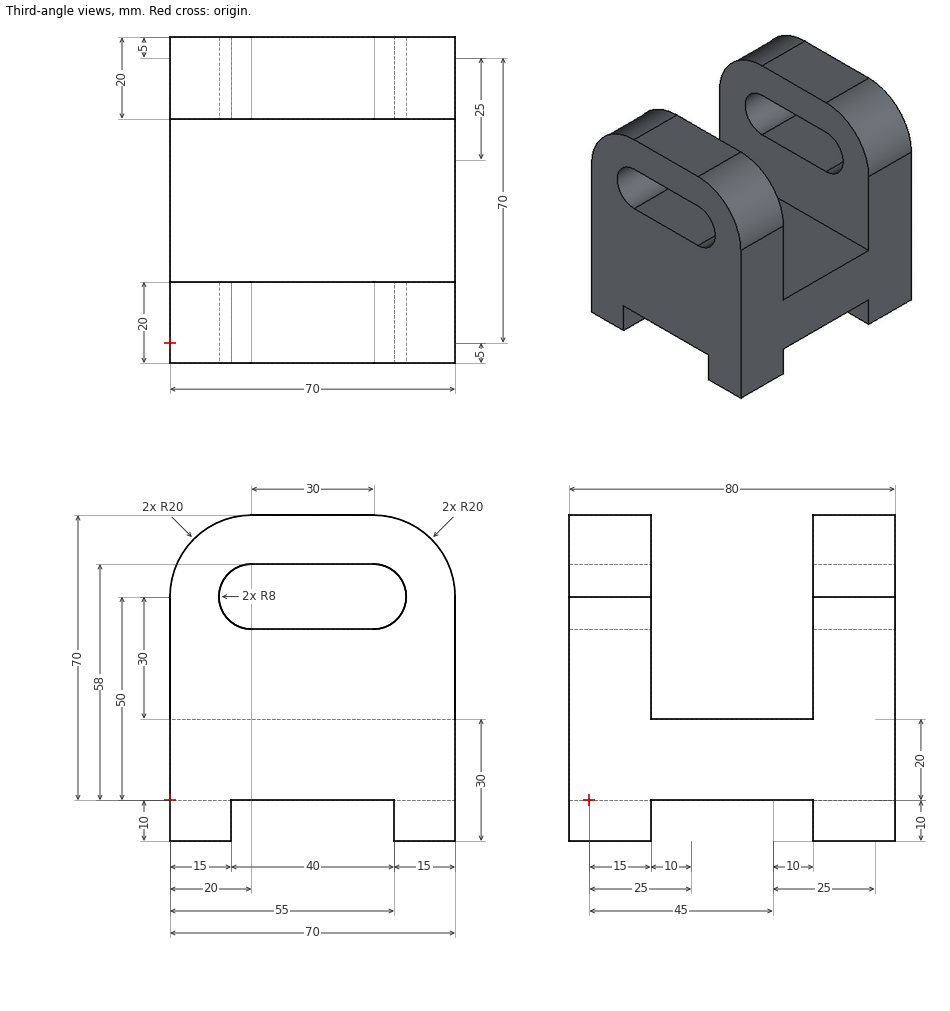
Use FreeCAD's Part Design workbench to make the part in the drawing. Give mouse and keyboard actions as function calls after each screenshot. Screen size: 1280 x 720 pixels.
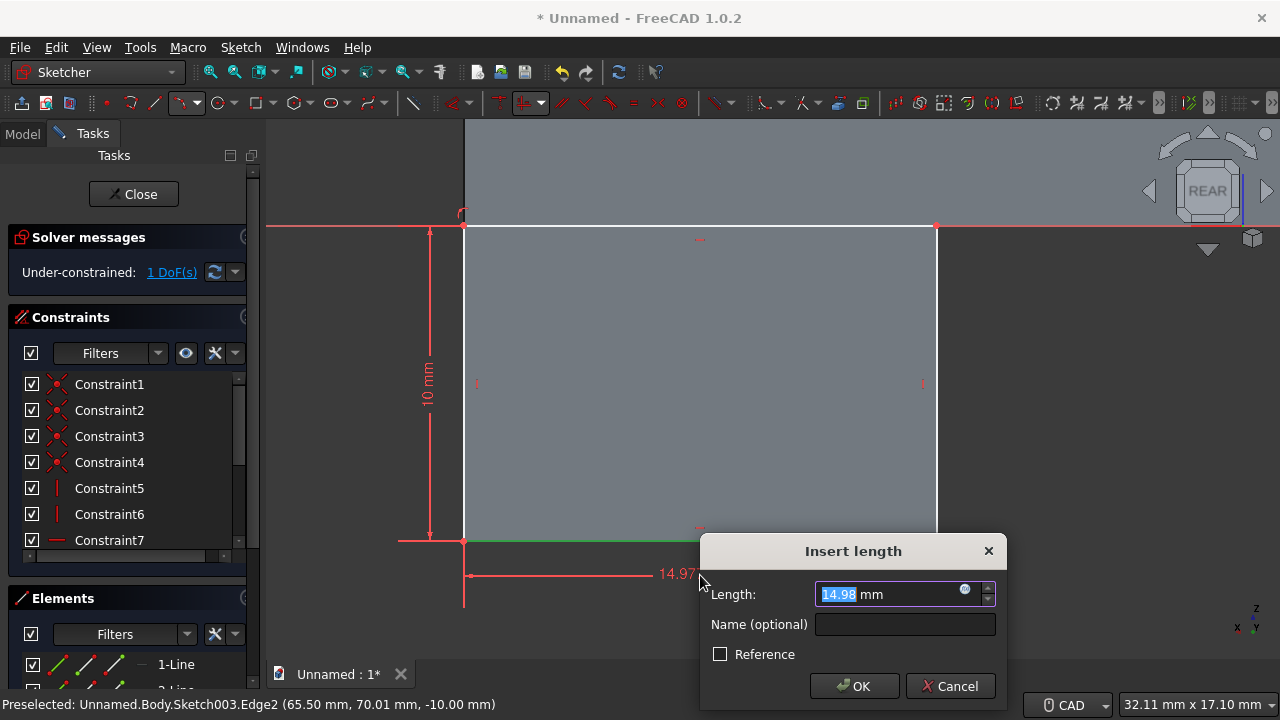
text(15)
key(Return)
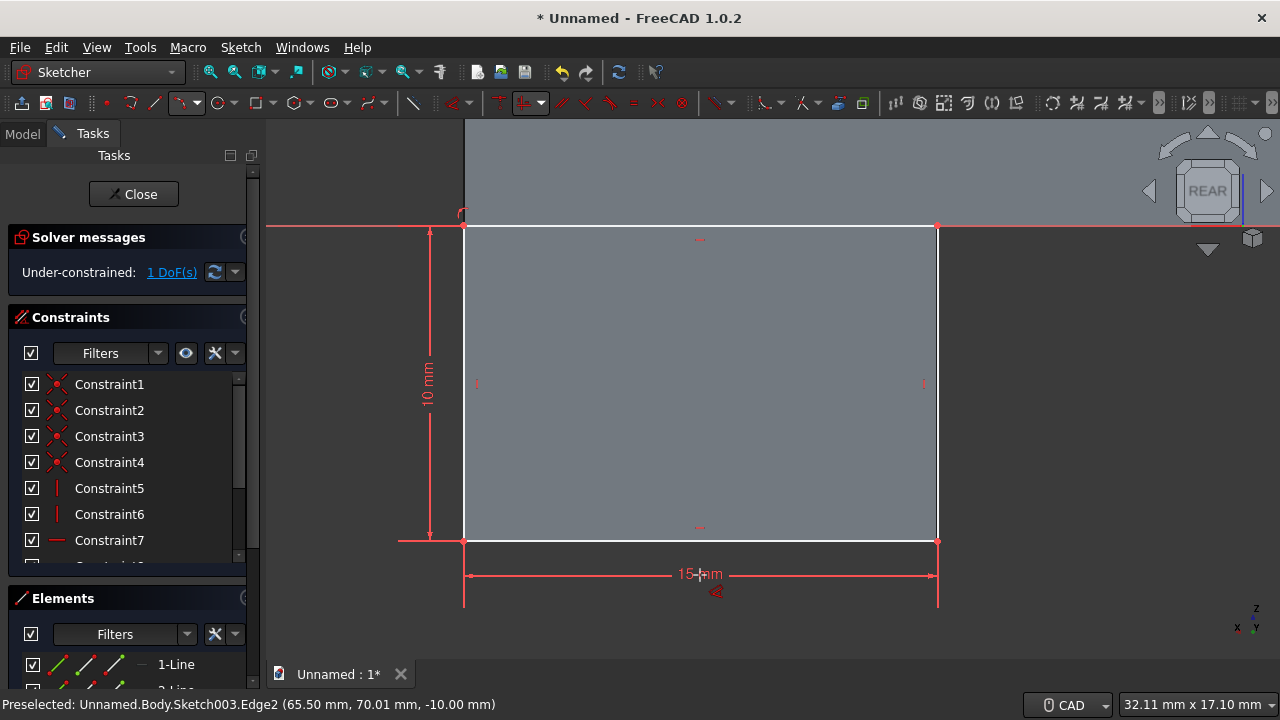
click(464, 226)
click(789, 192)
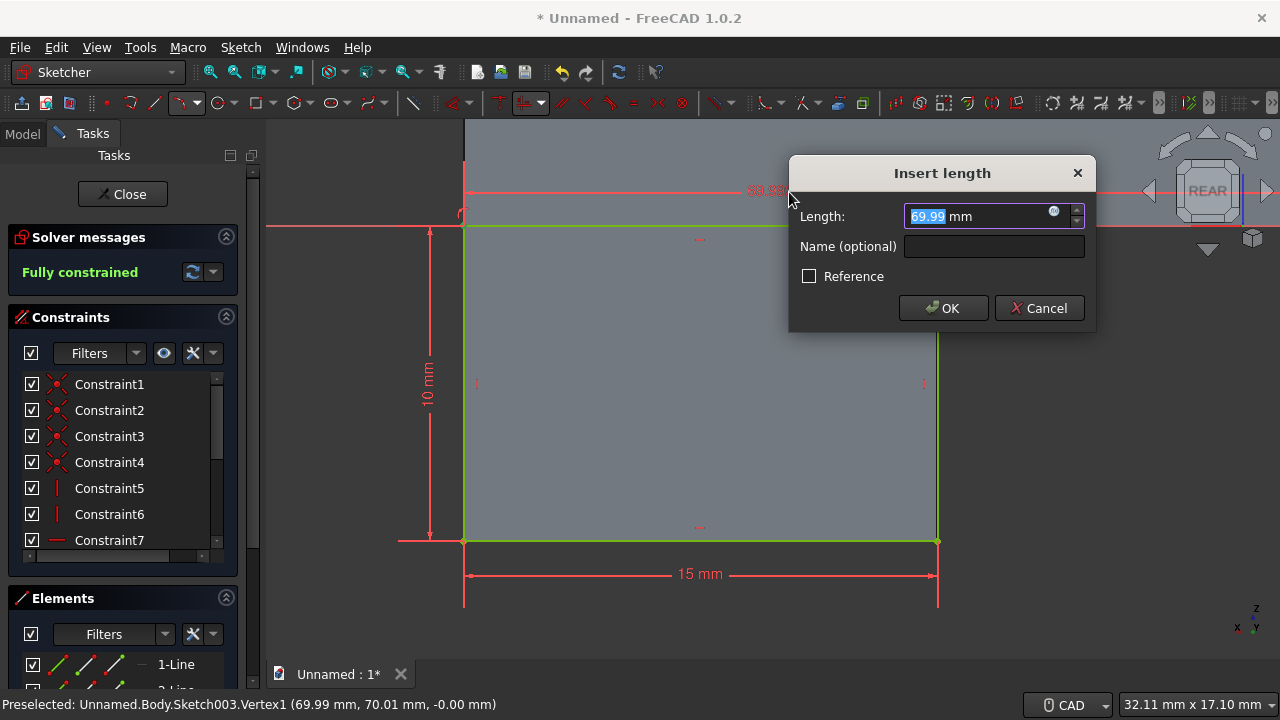
text(70)
key(Return)
key(Escape)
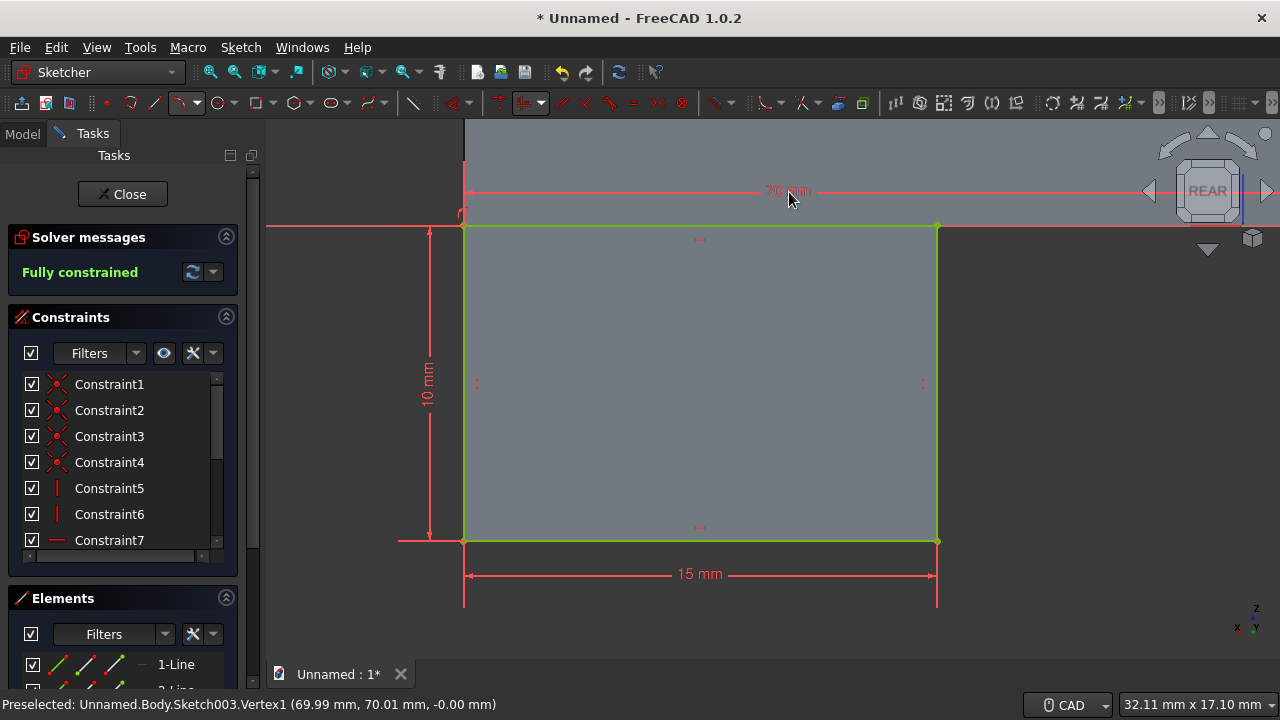
click(123, 194)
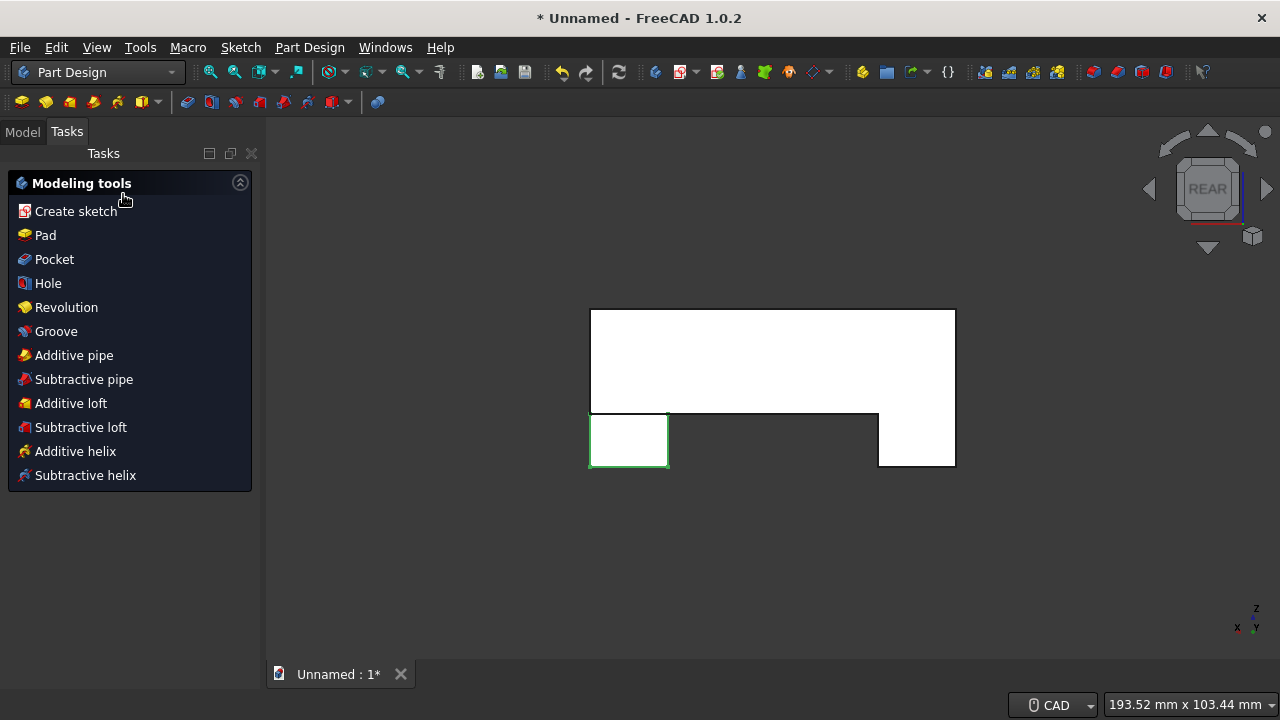
click(22, 102)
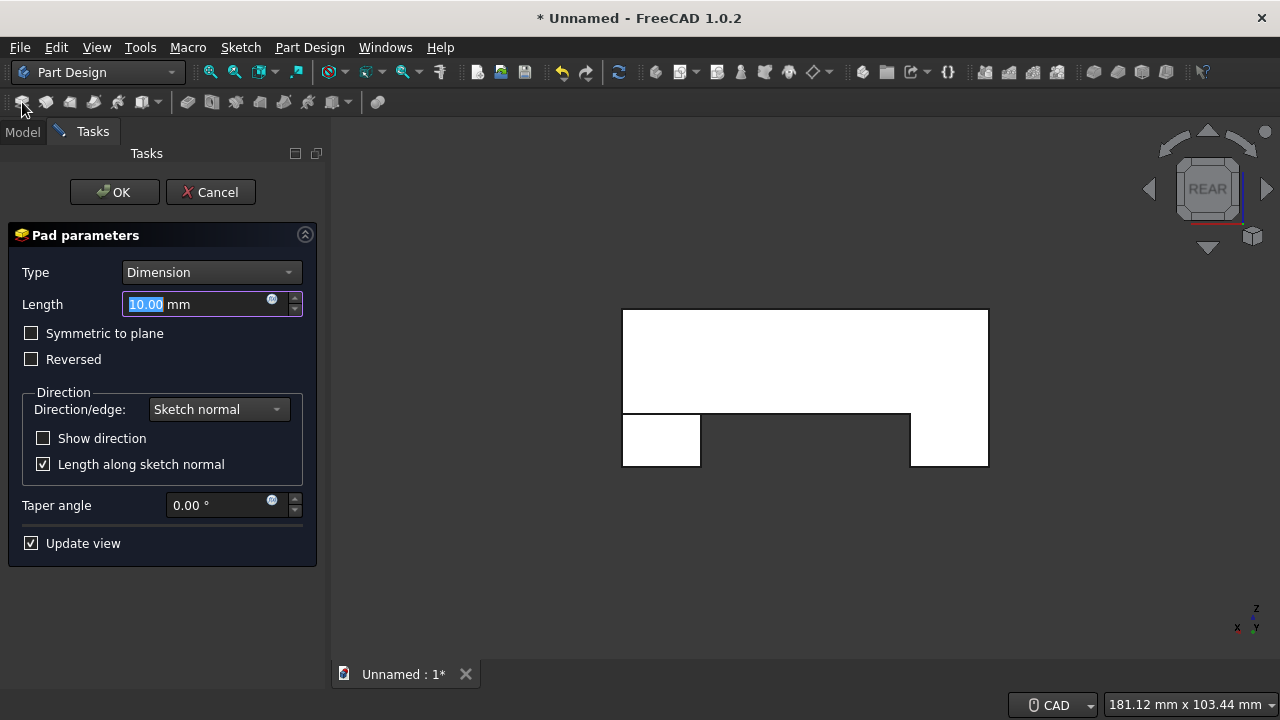
text(25)
key(Tab)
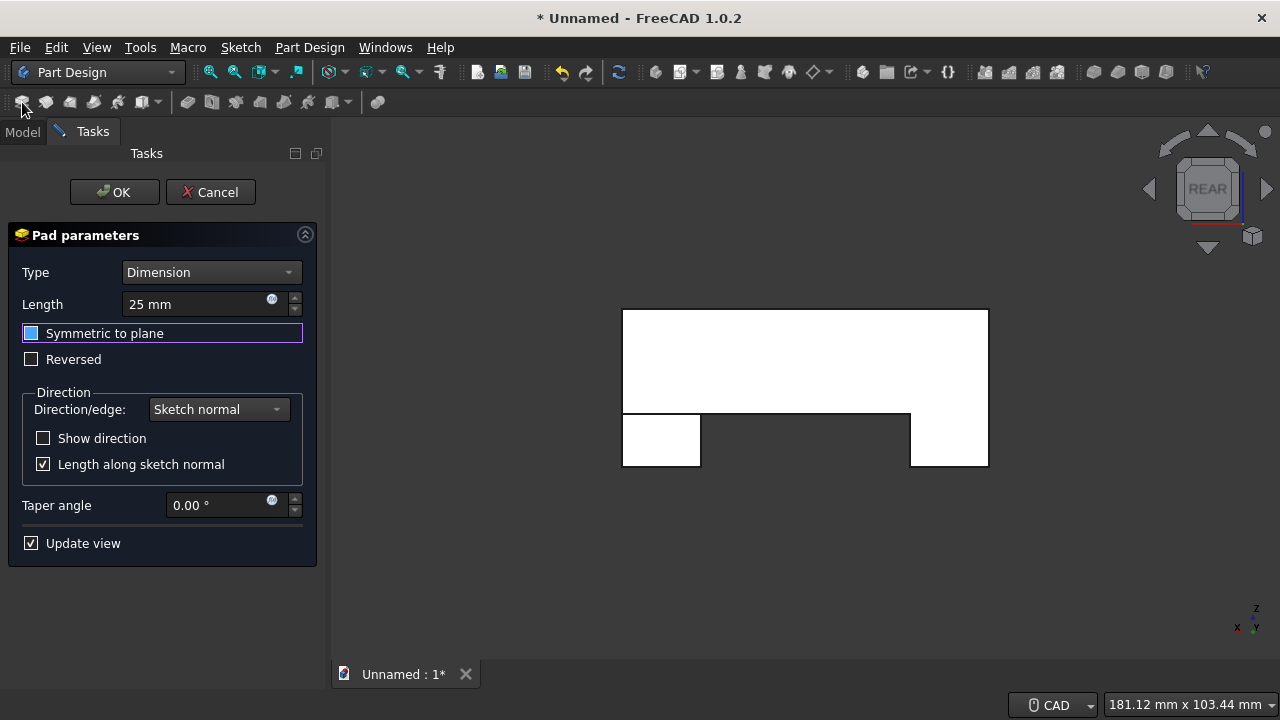
click(30, 359)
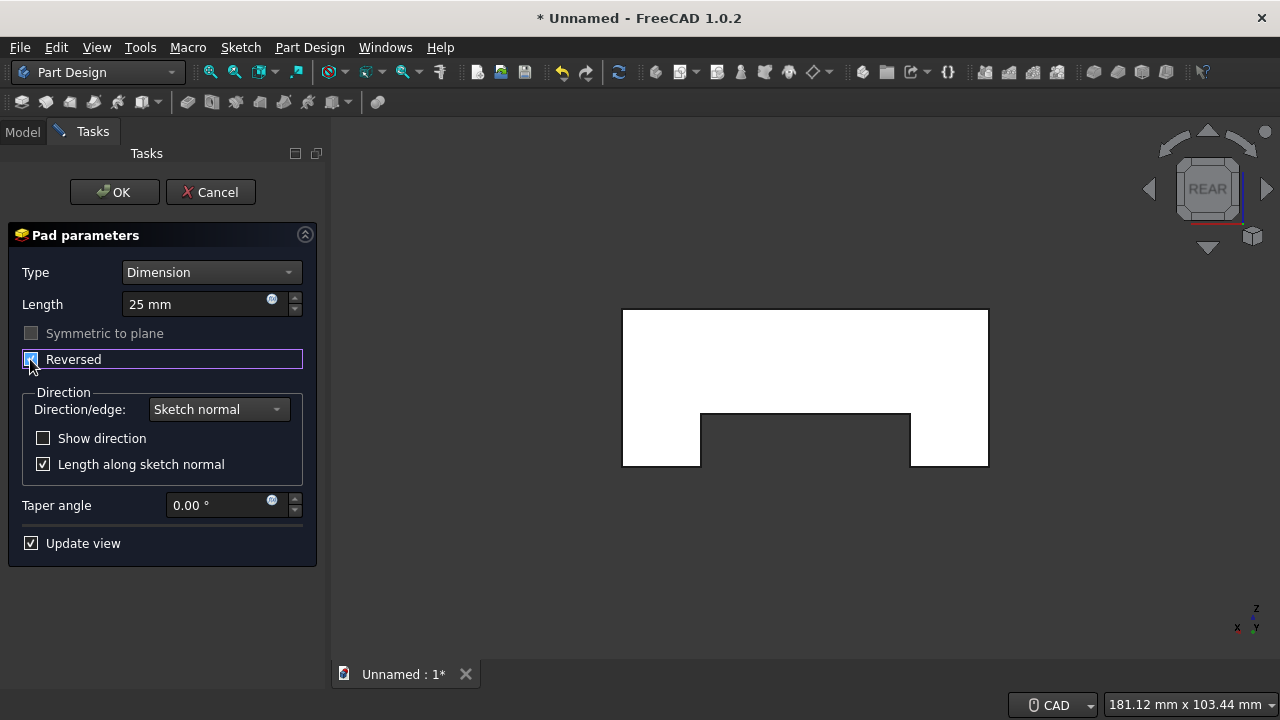
click(115, 192)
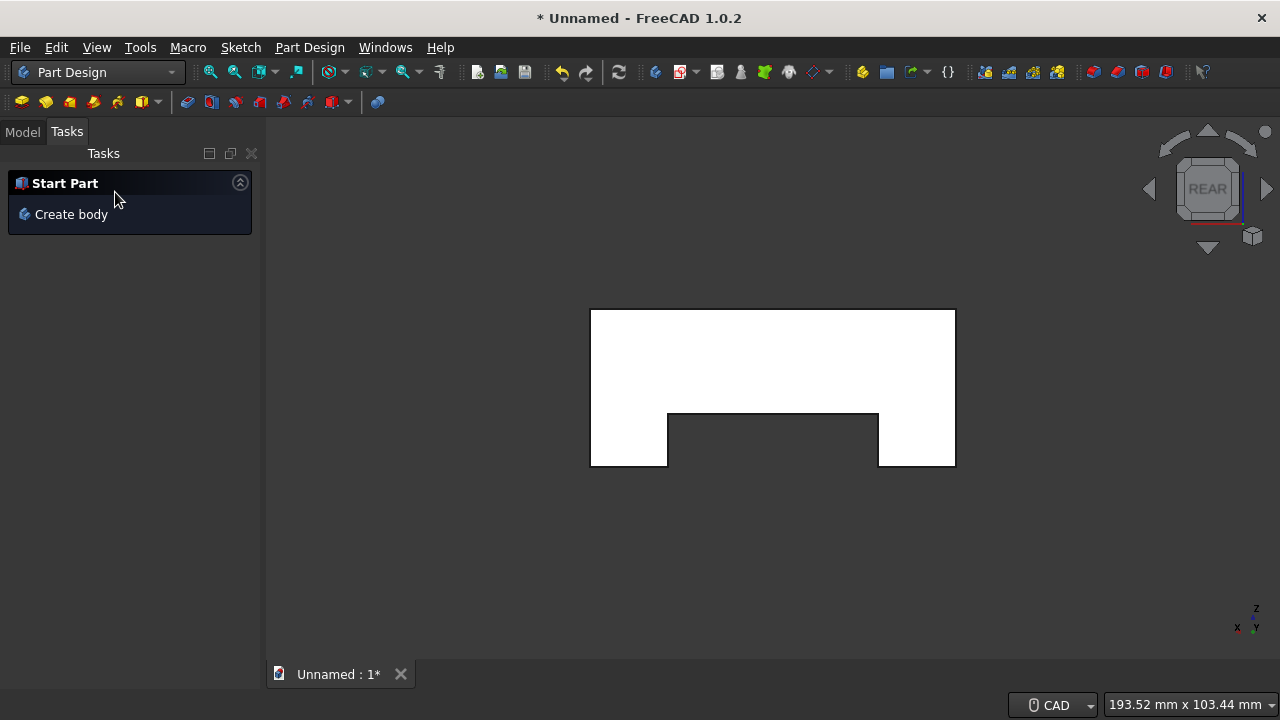
key(v)
key(f)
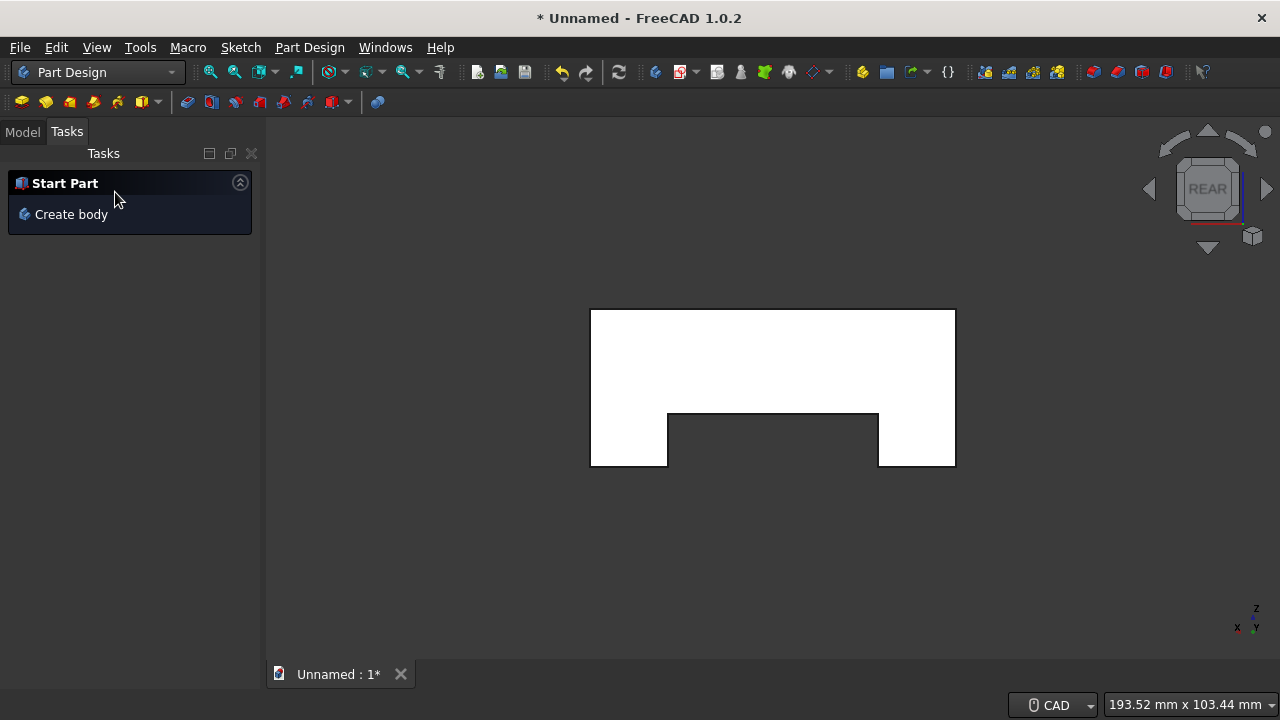
key(0)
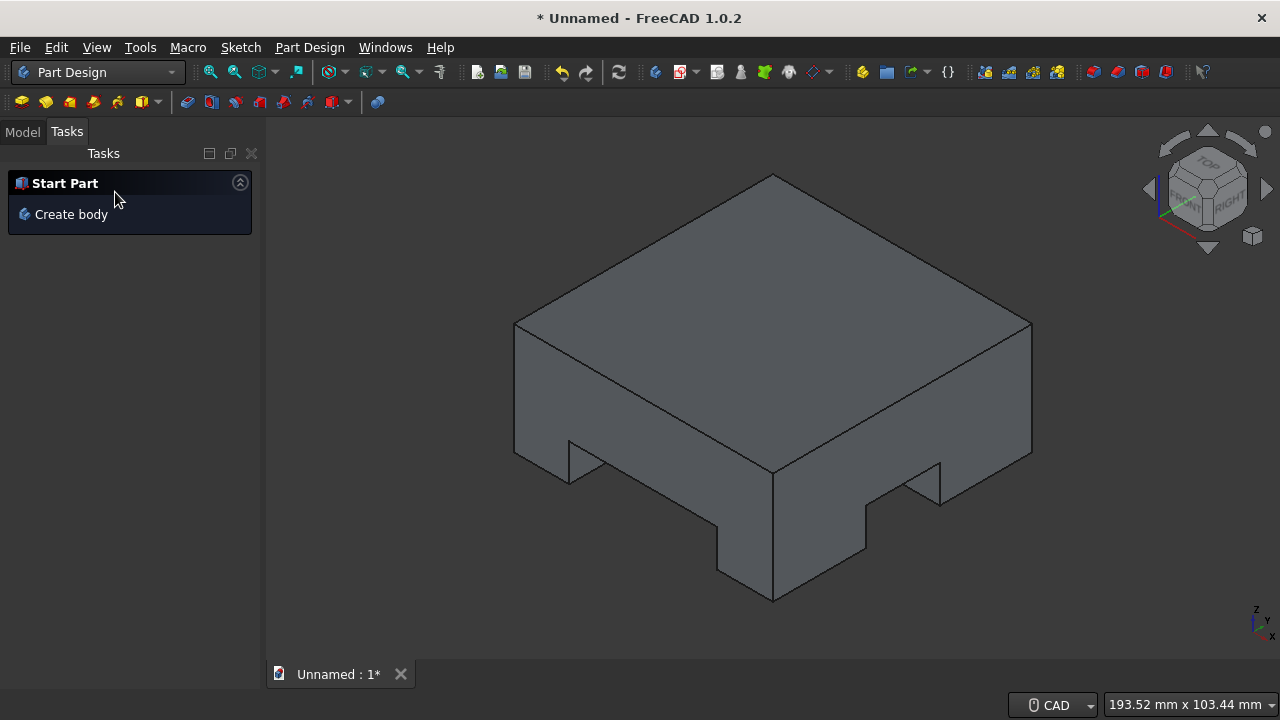
click(829, 505)